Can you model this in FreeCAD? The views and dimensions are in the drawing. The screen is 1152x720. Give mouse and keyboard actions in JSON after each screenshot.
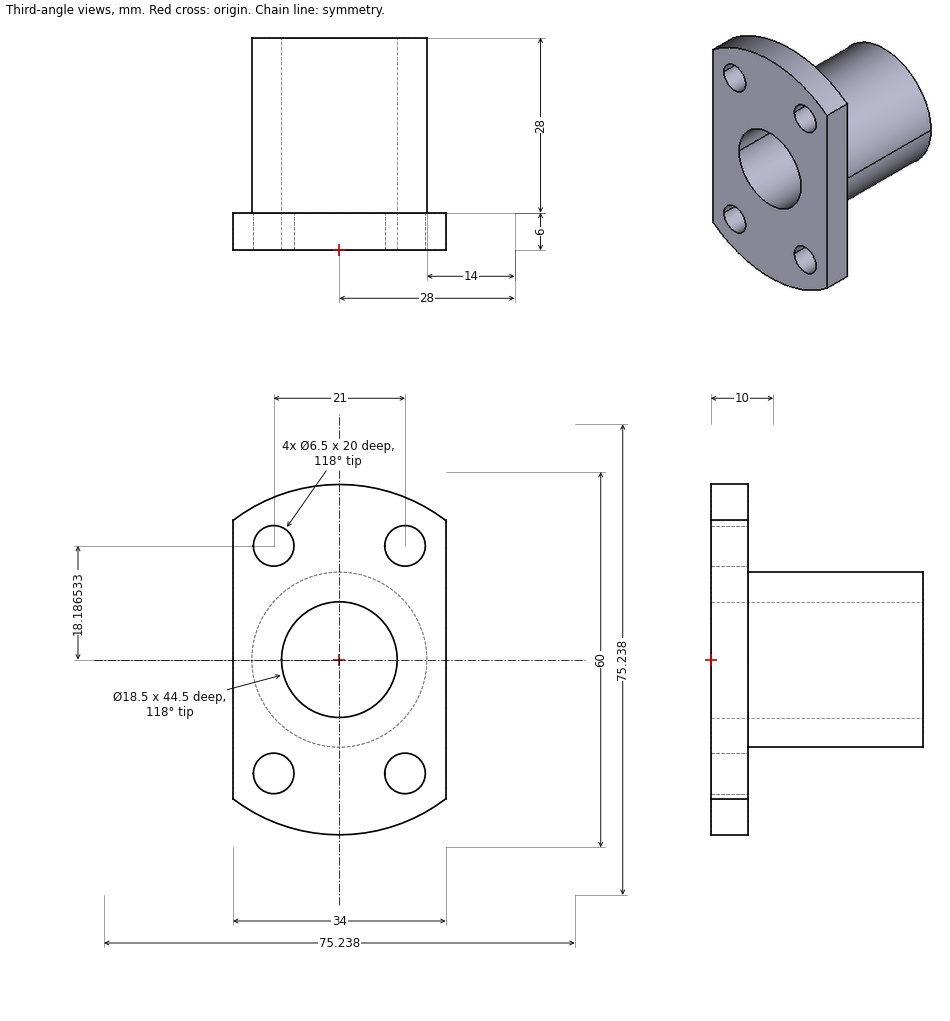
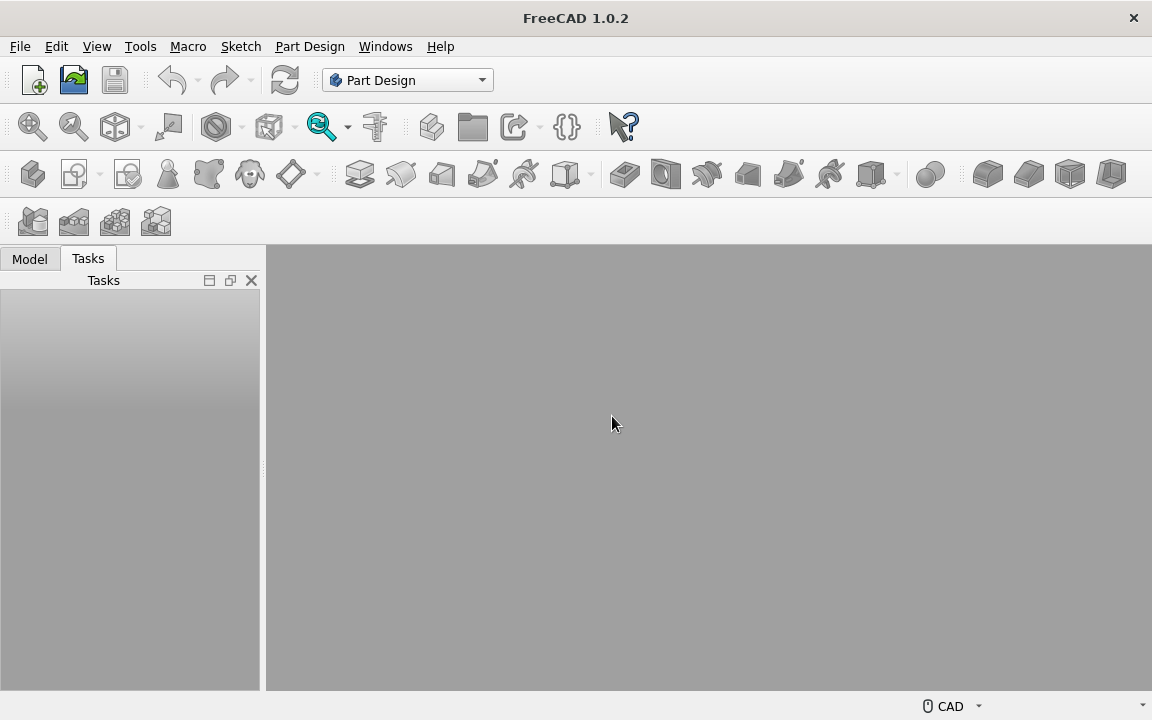
{"action": "left_click", "coordinate": [33, 80]}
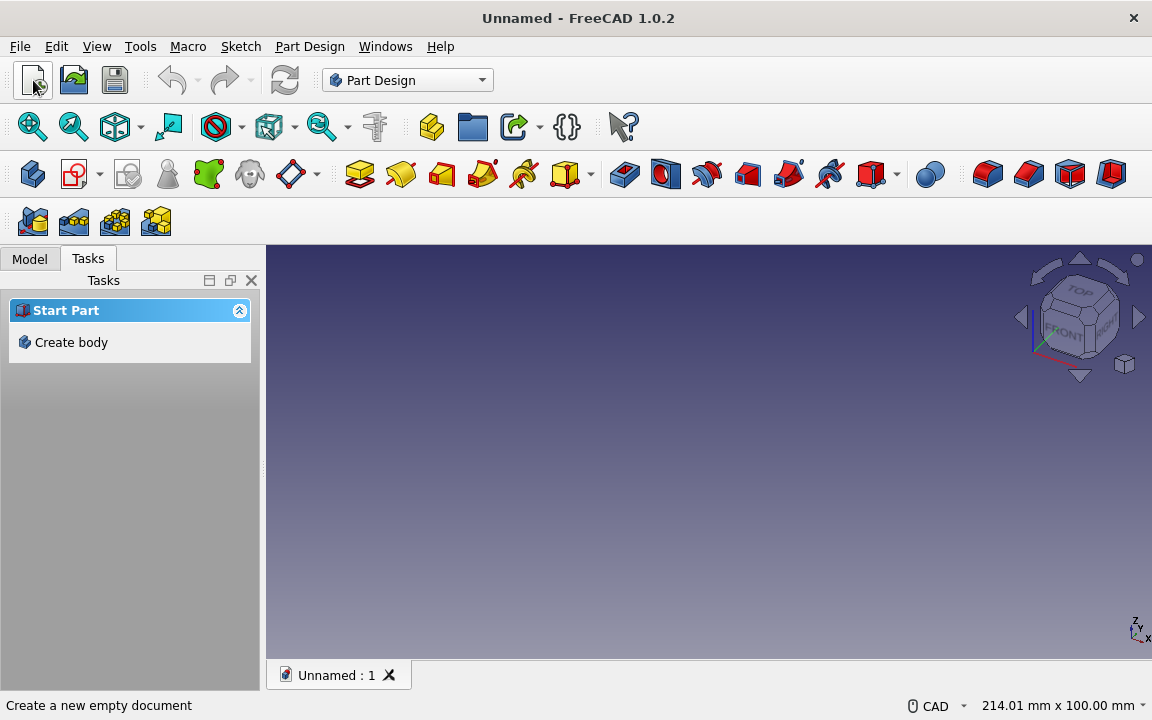
{"action": "left_click", "coordinate": [74, 174]}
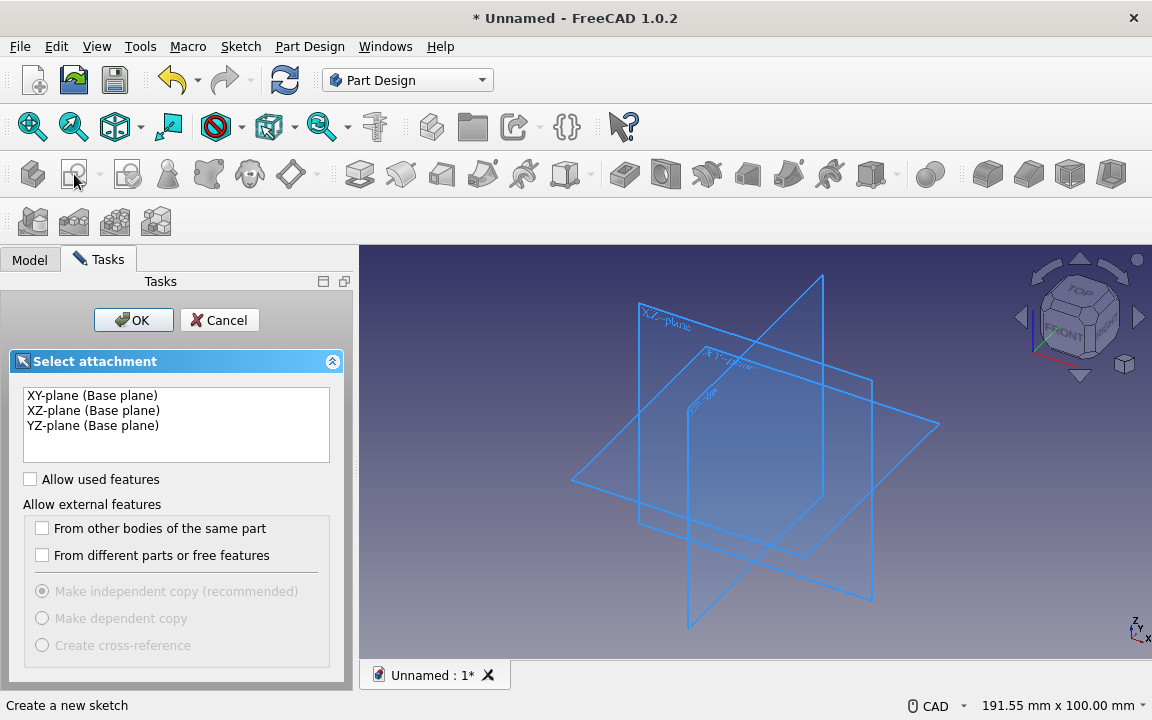
{"action": "left_click", "coordinate": [84, 396]}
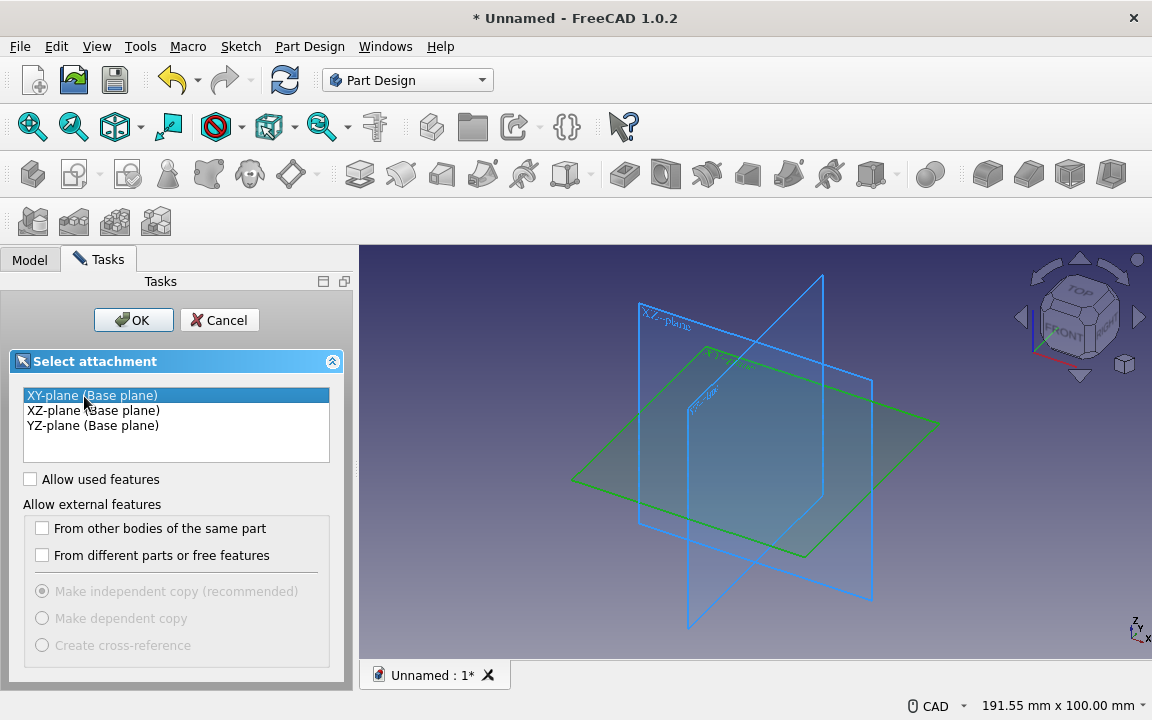
{"action": "left_click", "coordinate": [134, 320]}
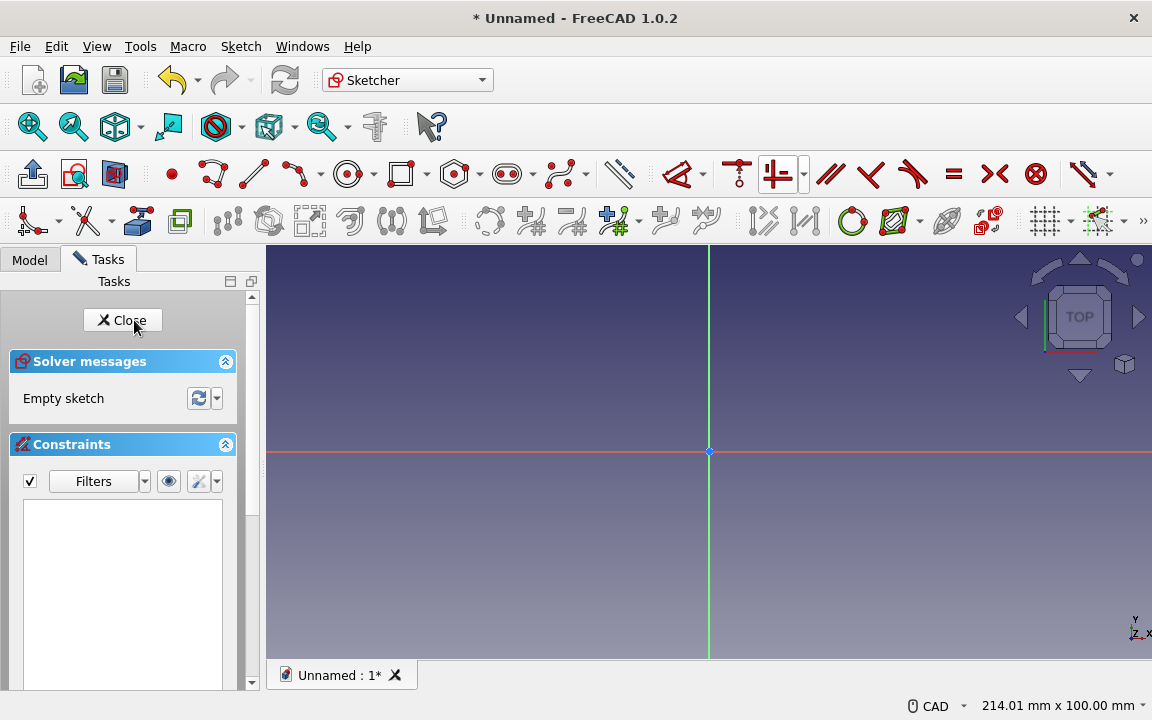
{"action": "scroll", "coordinate": [921, 296], "scroll_direction": "up", "scroll_amount": 3}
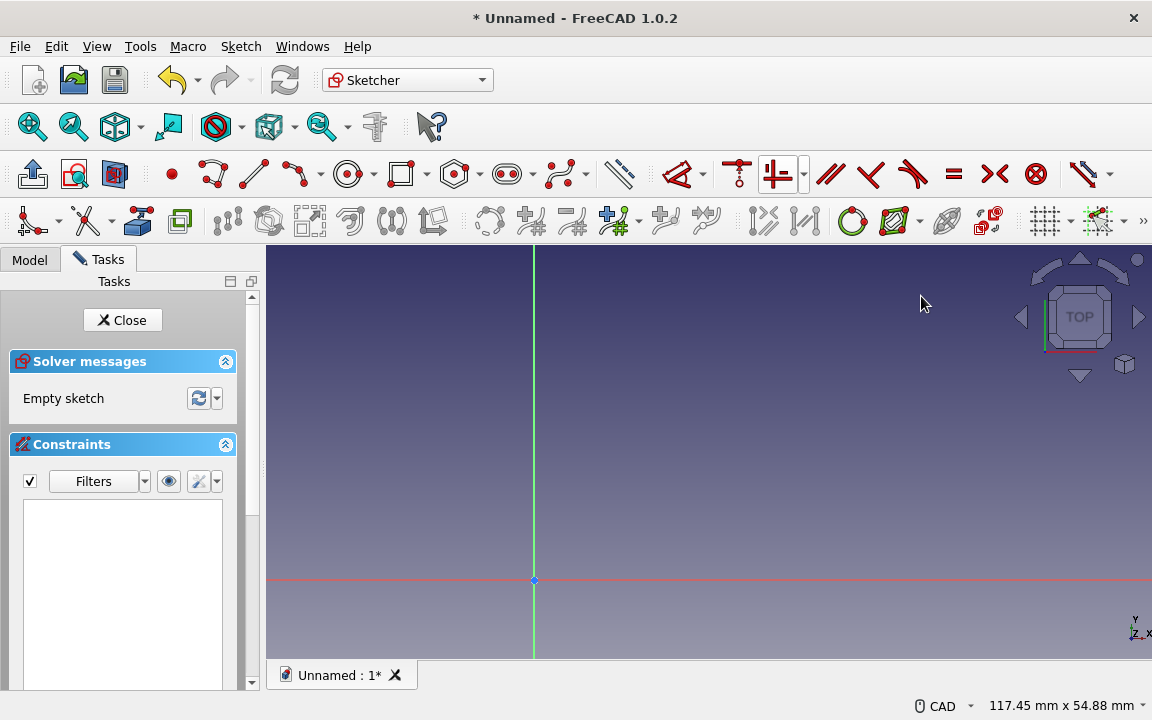
{"action": "left_click", "coordinate": [213, 174]}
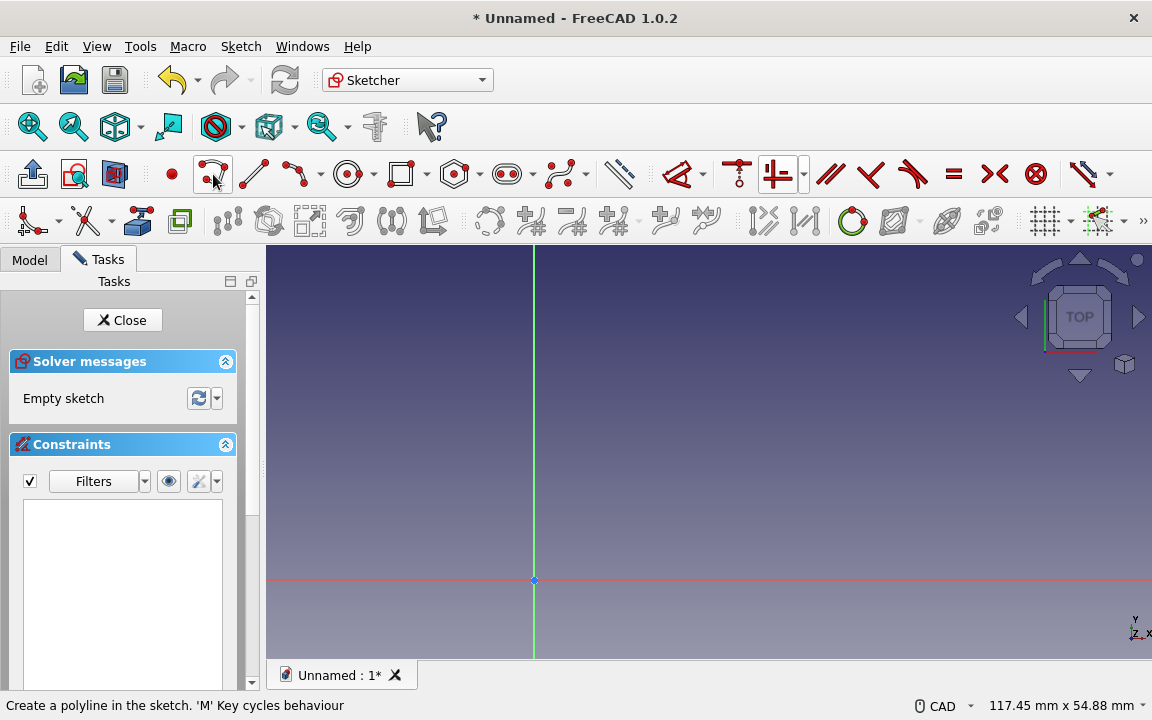
{"action": "left_click", "coordinate": [534, 580]}
{"action": "left_click", "coordinate": [745, 571]}
{"action": "left_click", "coordinate": [745, 535]}
{"action": "left_click", "coordinate": [640, 535]}
{"action": "left_click", "coordinate": [640, 324]}
{"action": "left_click", "coordinate": [543, 324]}
{"action": "left_click", "coordinate": [534, 580]}
{"action": "key", "text": "Escape"}
{"action": "key", "text": "Escape"}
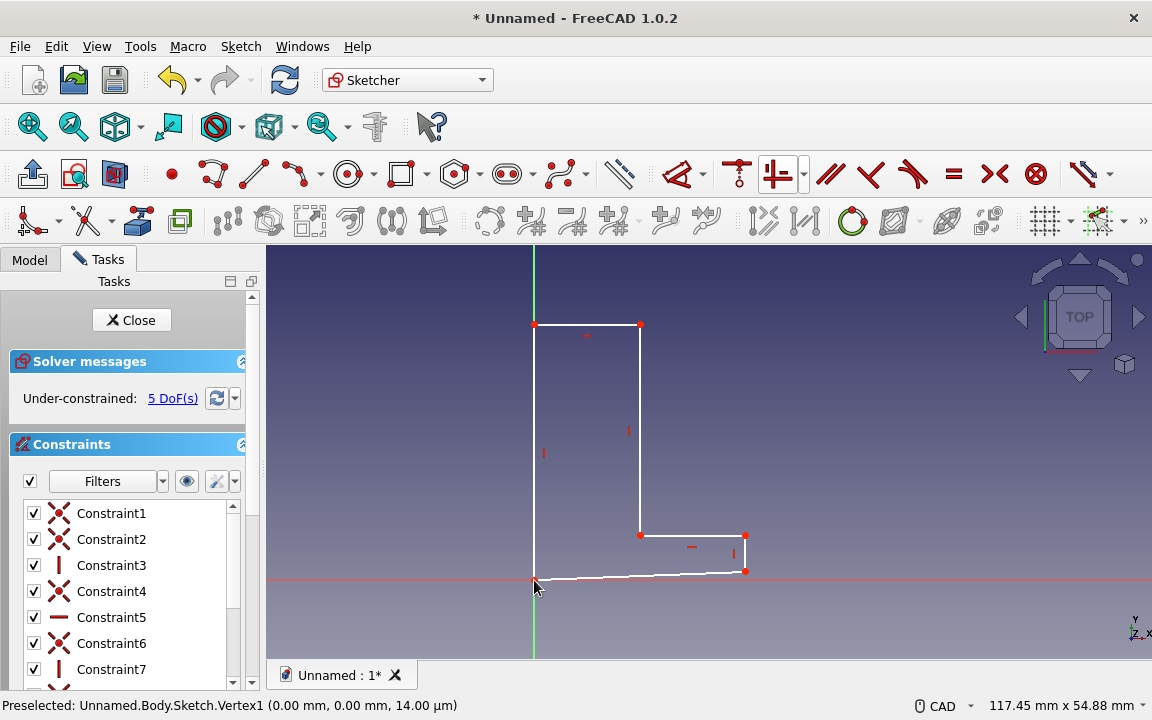
{"action": "left_click", "coordinate": [597, 578]}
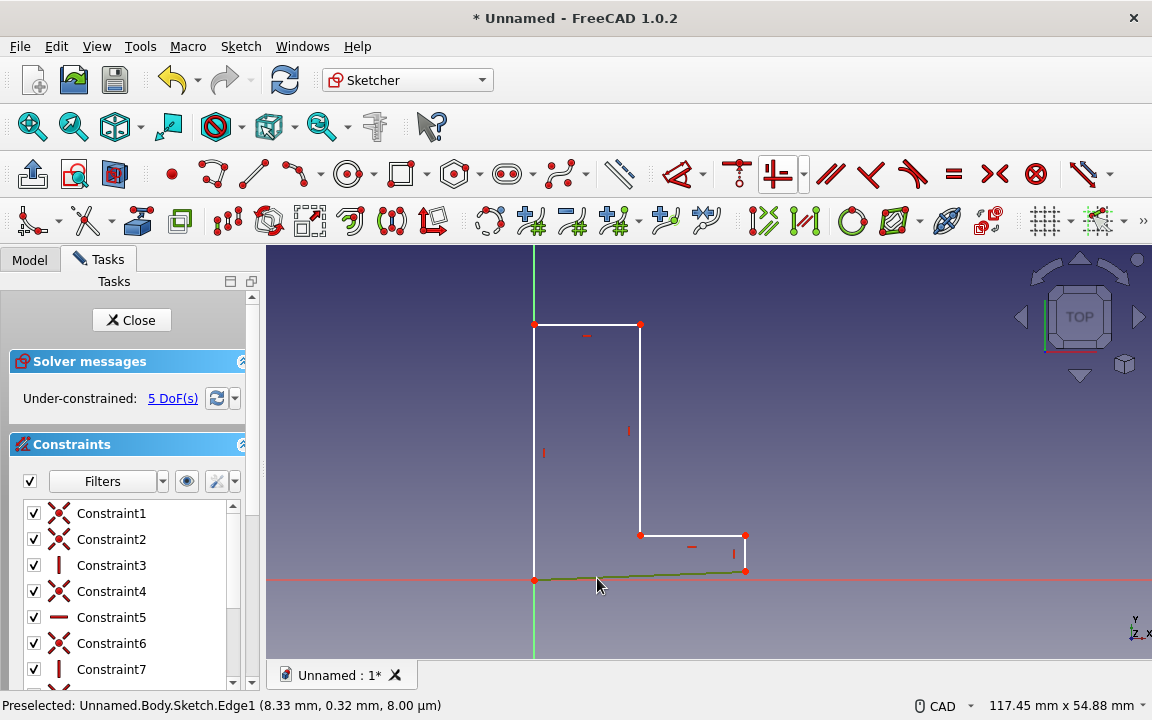
{"action": "key", "text": "h"}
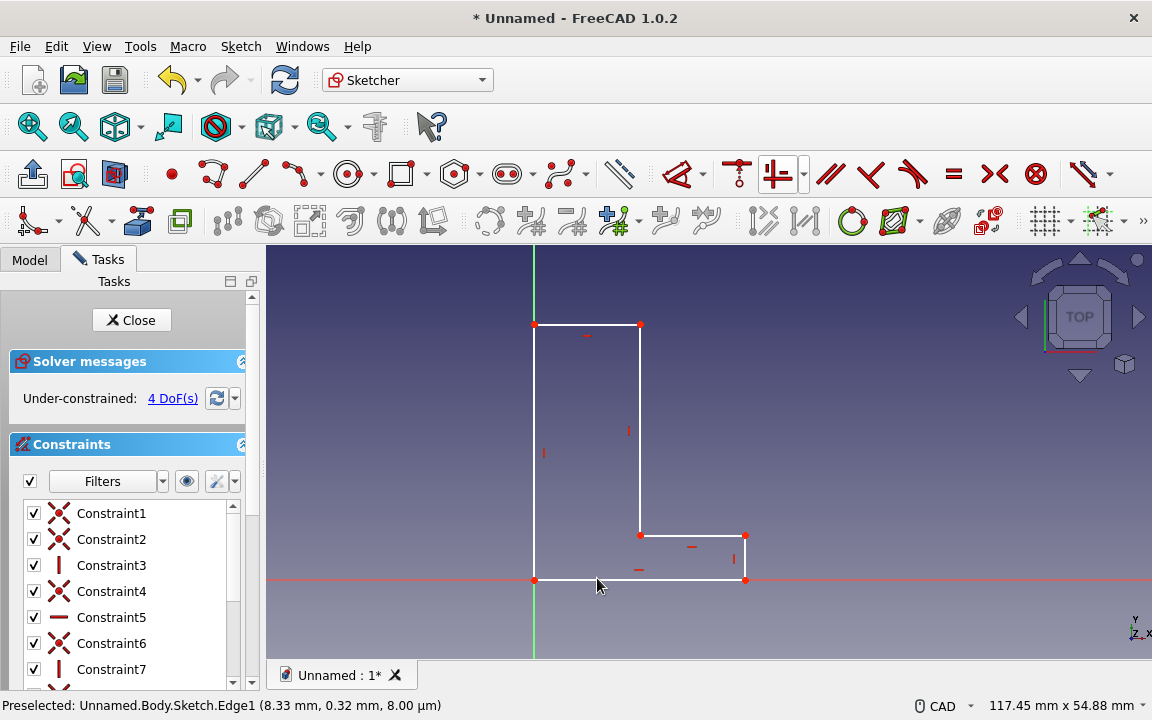
{"action": "left_click", "coordinate": [676, 174]}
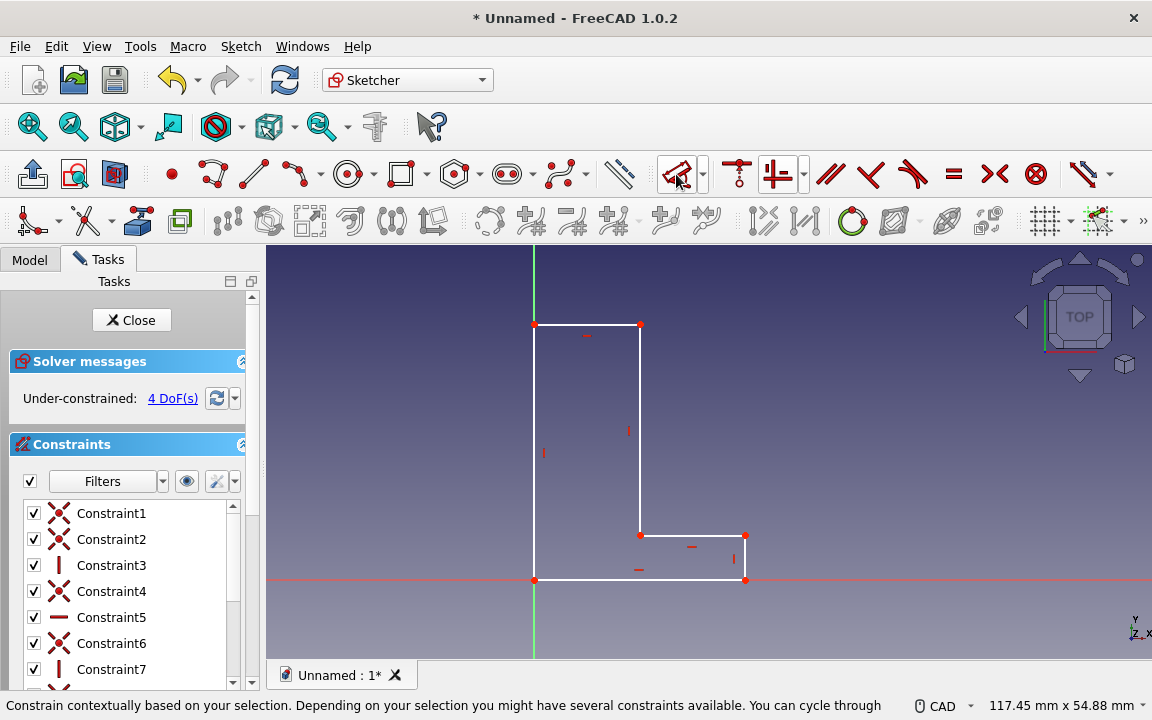
{"action": "left_click", "coordinate": [745, 567]}
{"action": "left_click", "coordinate": [779, 558]}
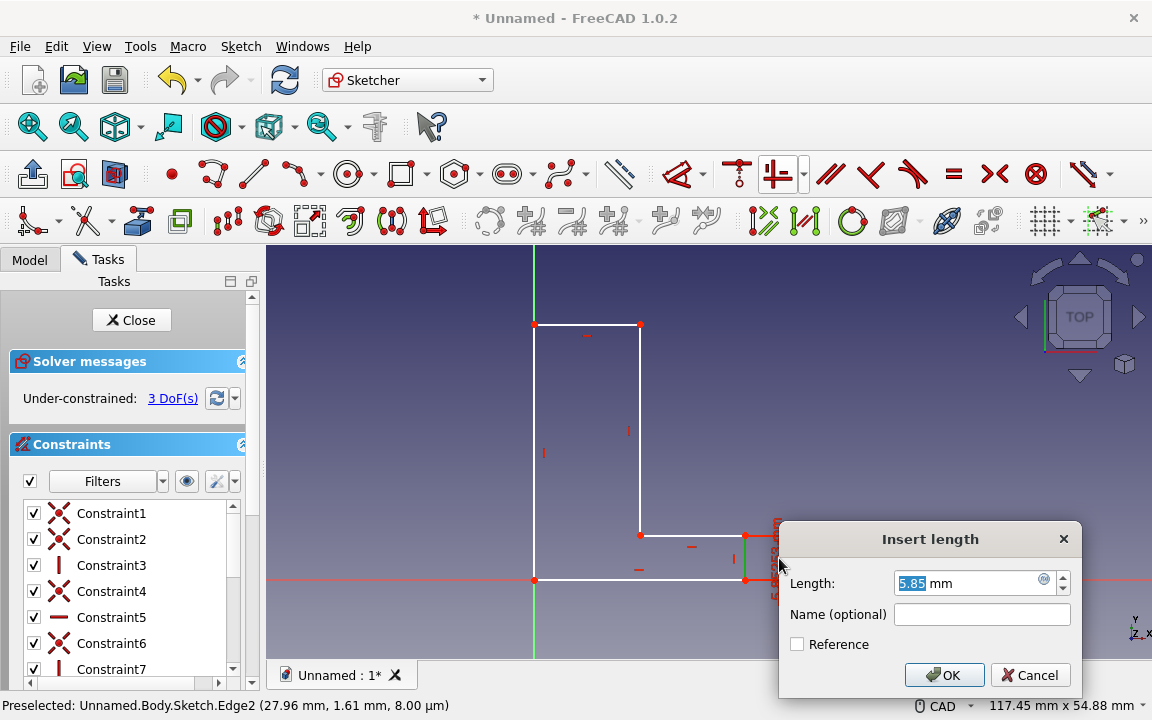
{"action": "type", "text": "6"}
{"action": "key", "text": "Return"}